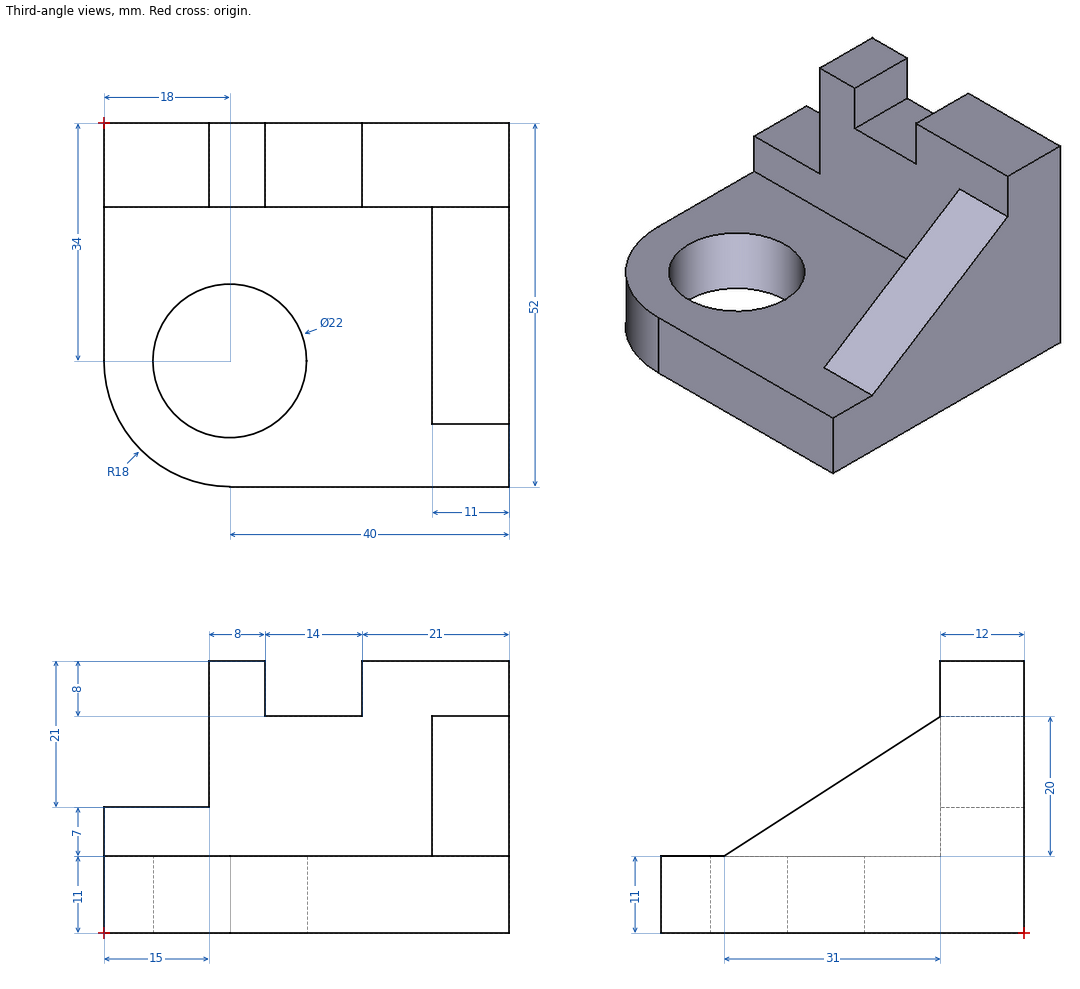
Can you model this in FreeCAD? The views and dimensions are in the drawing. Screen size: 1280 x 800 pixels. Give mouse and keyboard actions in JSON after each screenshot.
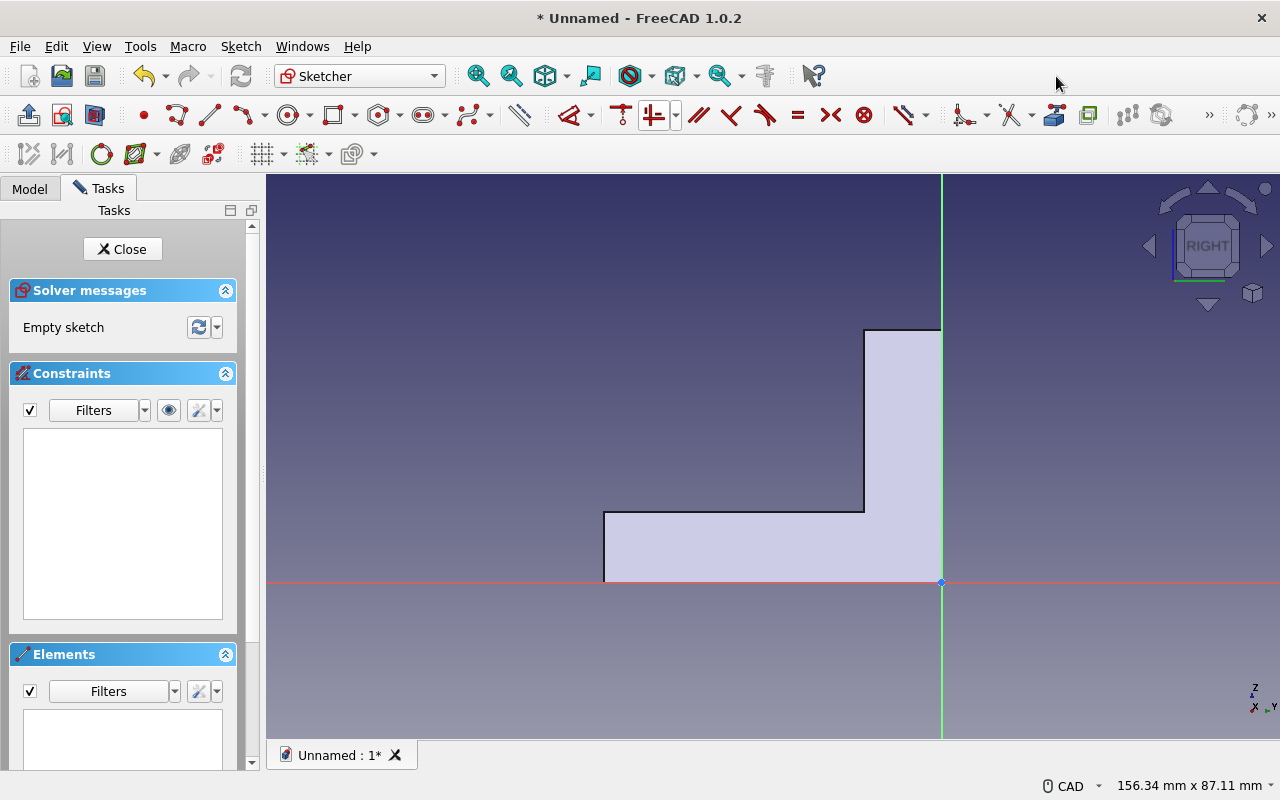
{"action": "scroll", "coordinate": [921, 514], "scroll_direction": "up", "scroll_amount": 3}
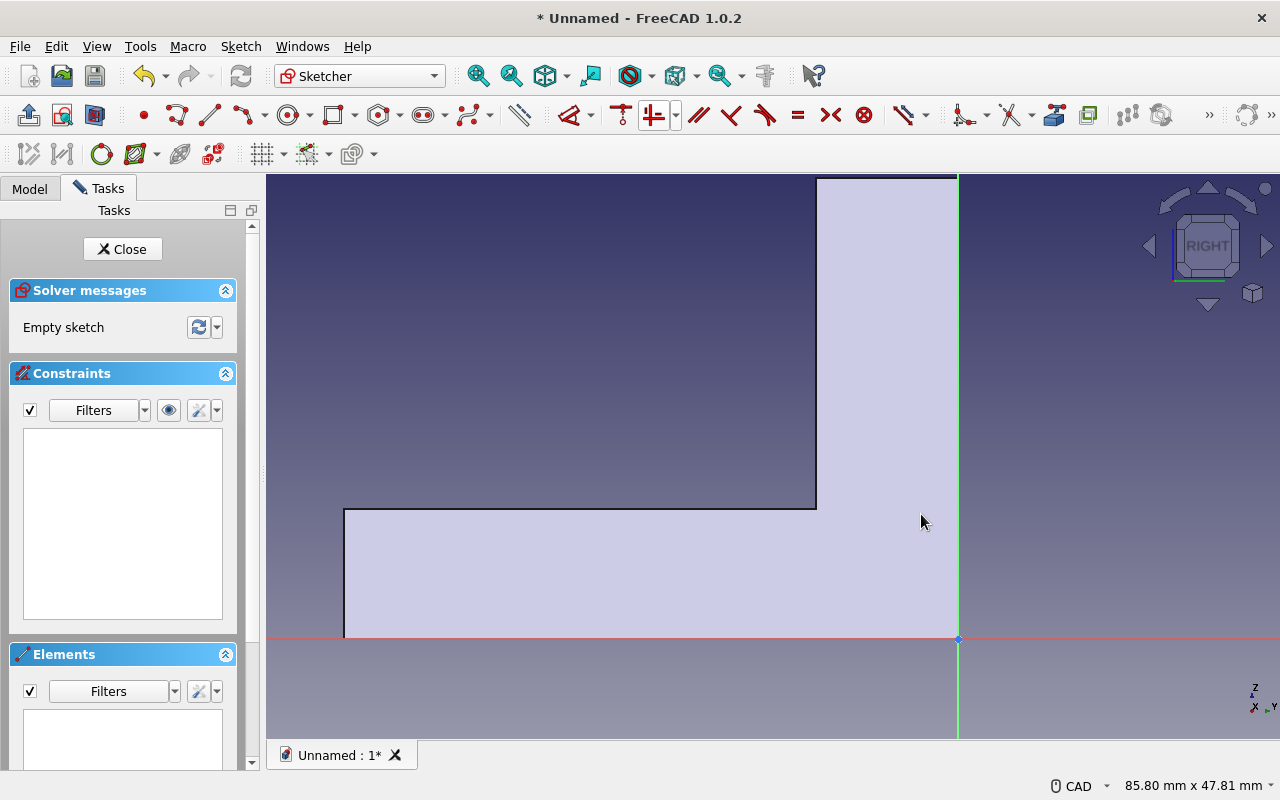
{"action": "left_click", "coordinate": [177, 116]}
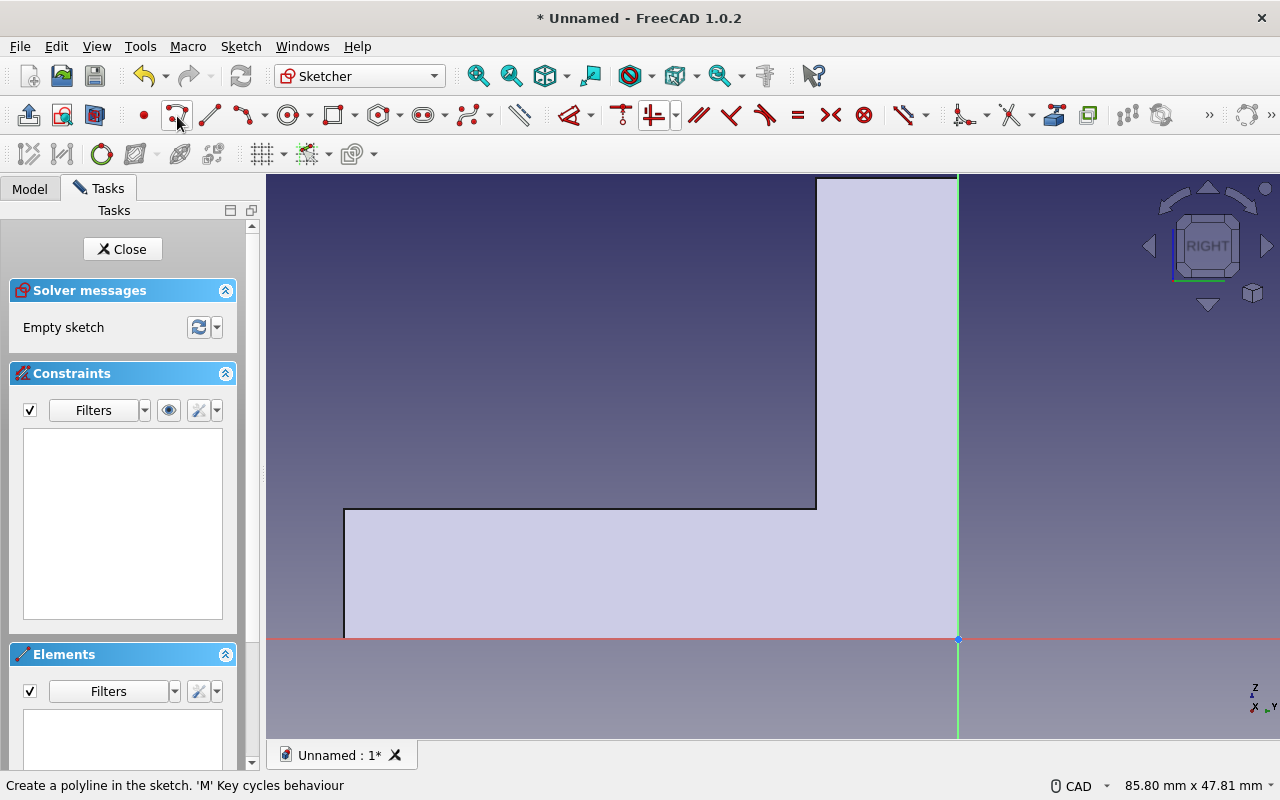
{"action": "left_click", "coordinate": [816, 509]}
{"action": "left_click", "coordinate": [816, 273]}
{"action": "left_click", "coordinate": [450, 509]}
{"action": "left_click", "coordinate": [816, 510]}
{"action": "key", "text": "Escape"}
{"action": "key", "text": "Escape"}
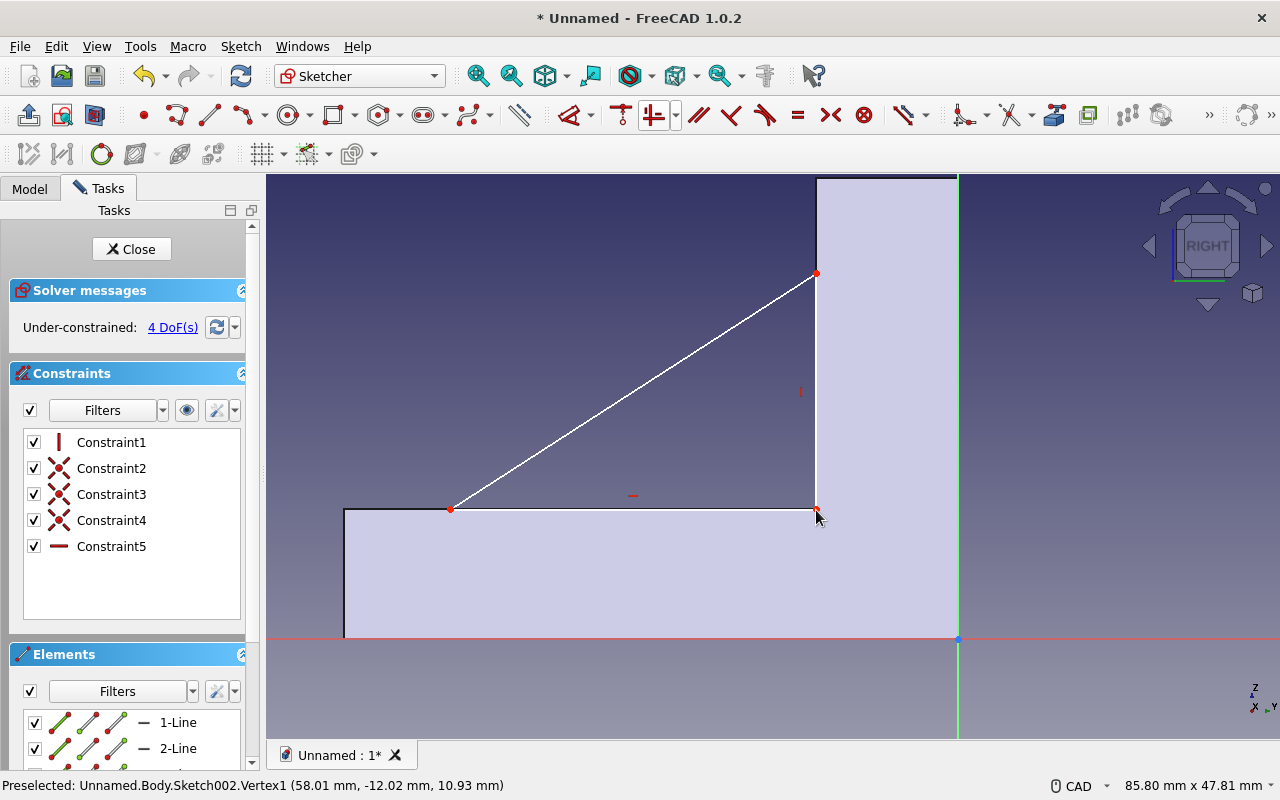
{"action": "left_click", "coordinate": [568, 116]}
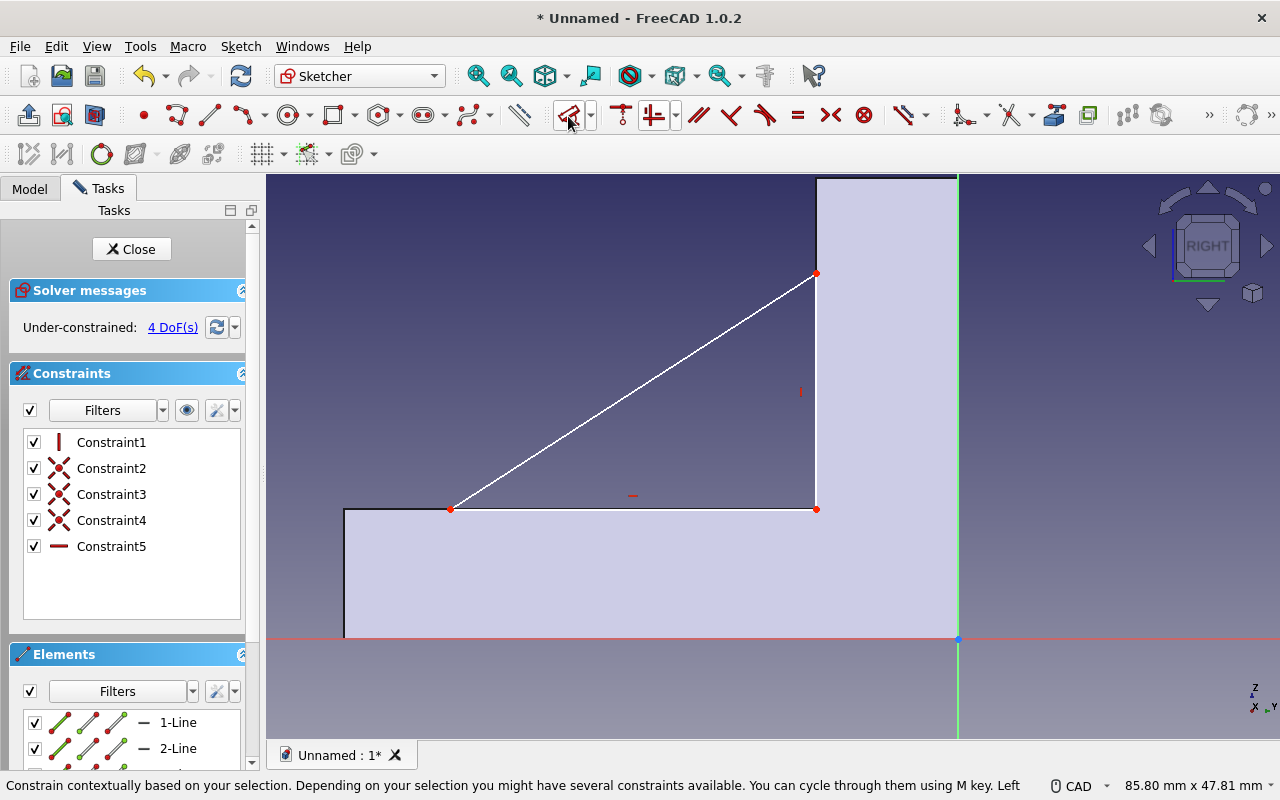
{"action": "left_click", "coordinate": [816, 439]}
{"action": "left_click", "coordinate": [850, 392]}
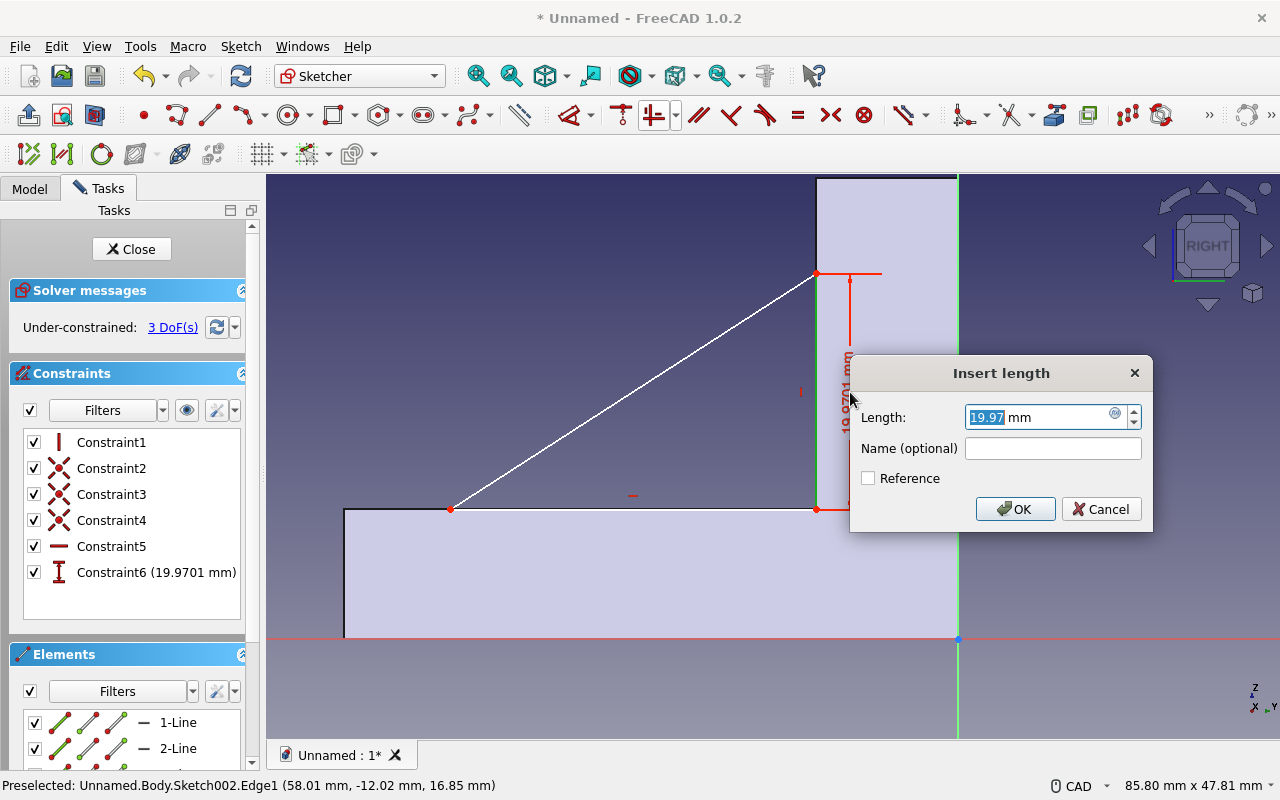
{"action": "type", "text": "20"}
{"action": "key", "text": "Return"}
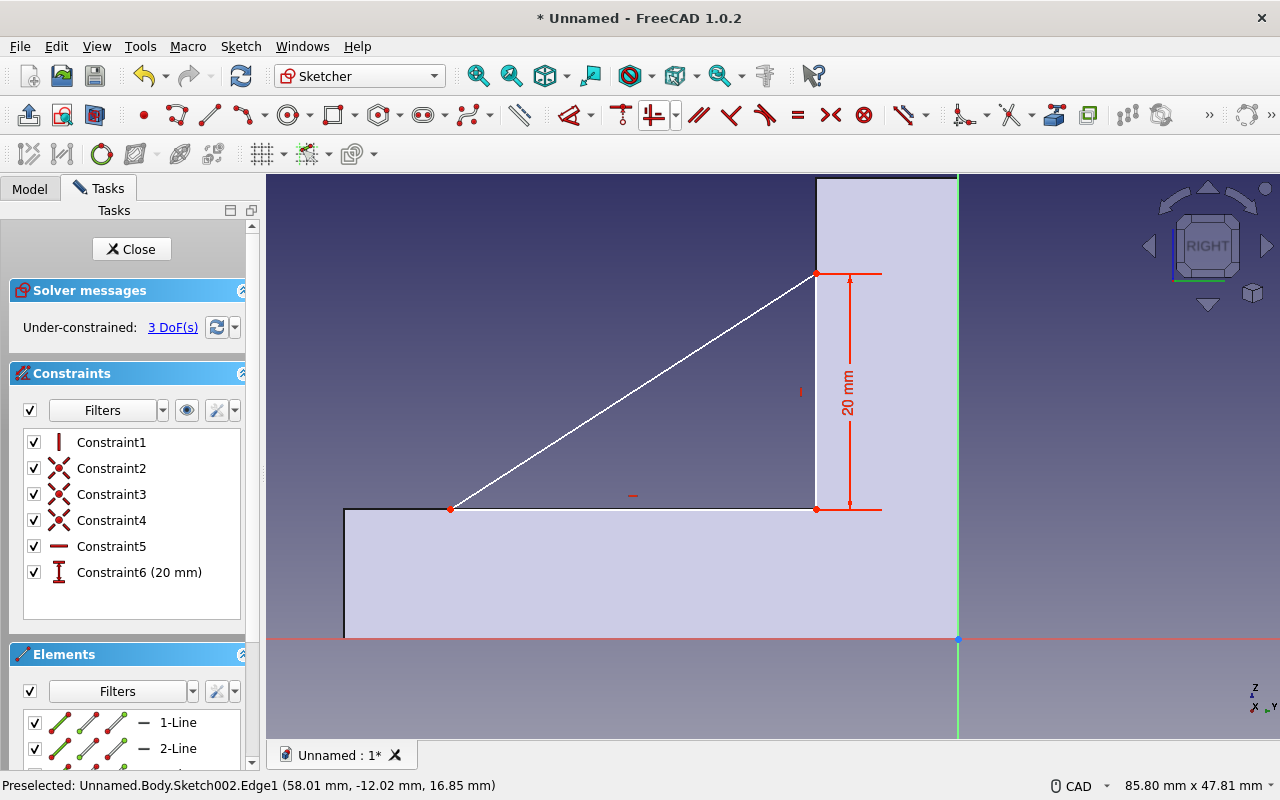
{"action": "left_click", "coordinate": [560, 510]}
{"action": "left_click", "coordinate": [633, 544]}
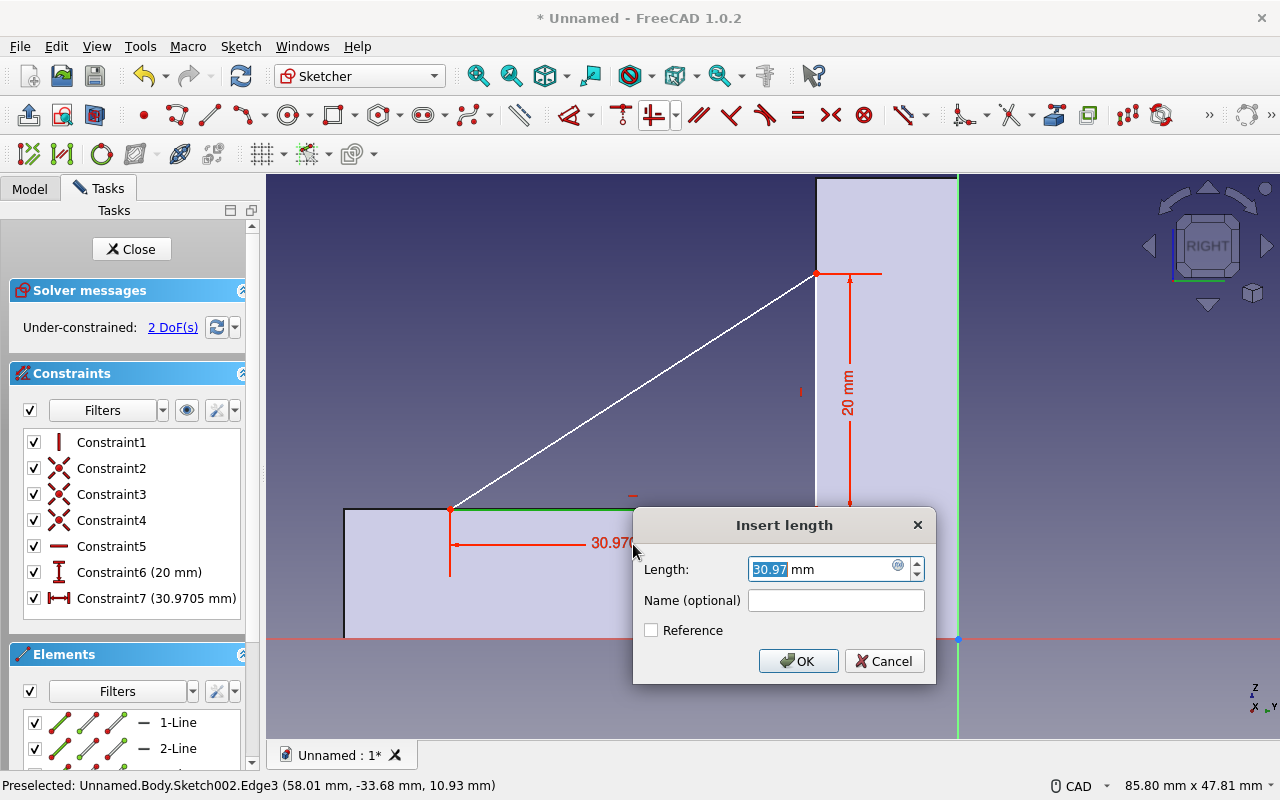
{"action": "type", "text": "31"}
{"action": "key", "text": "Return"}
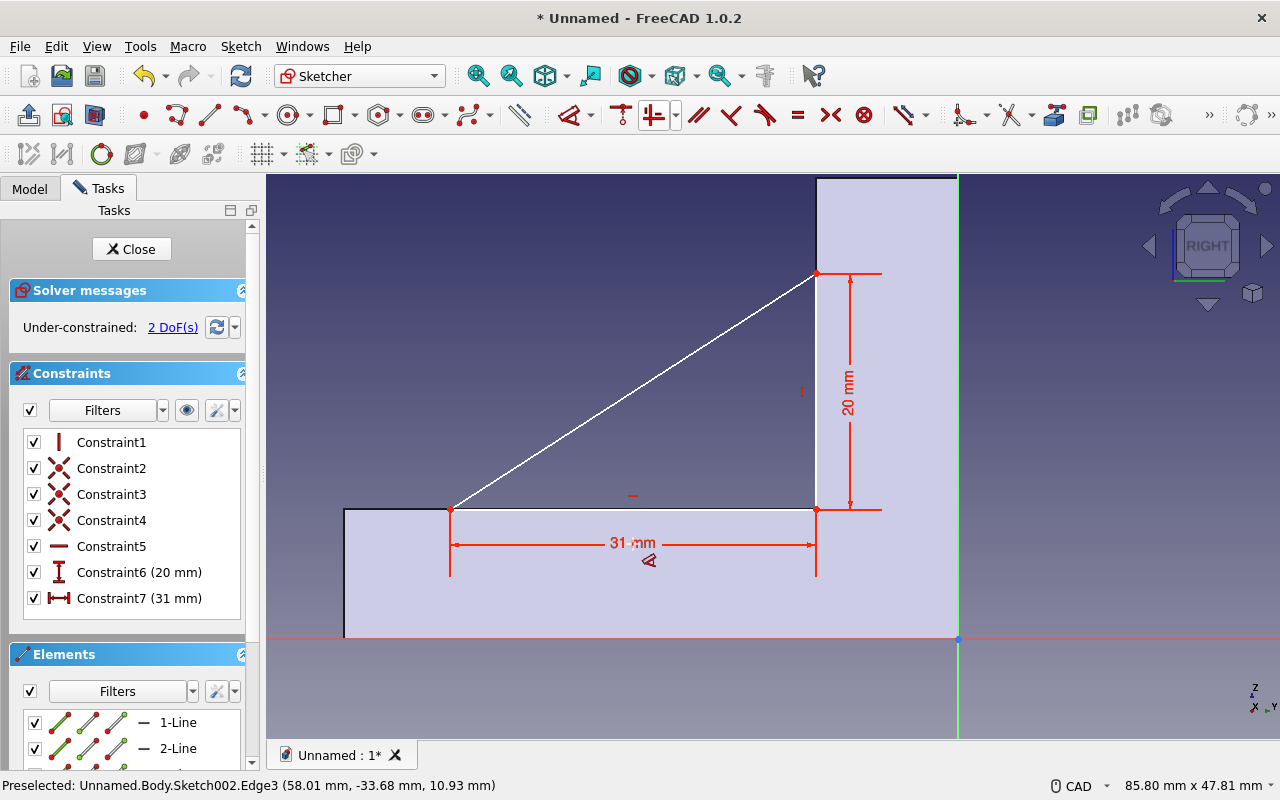
{"action": "left_click", "coordinate": [816, 510]}
{"action": "left_click", "coordinate": [887, 673]}